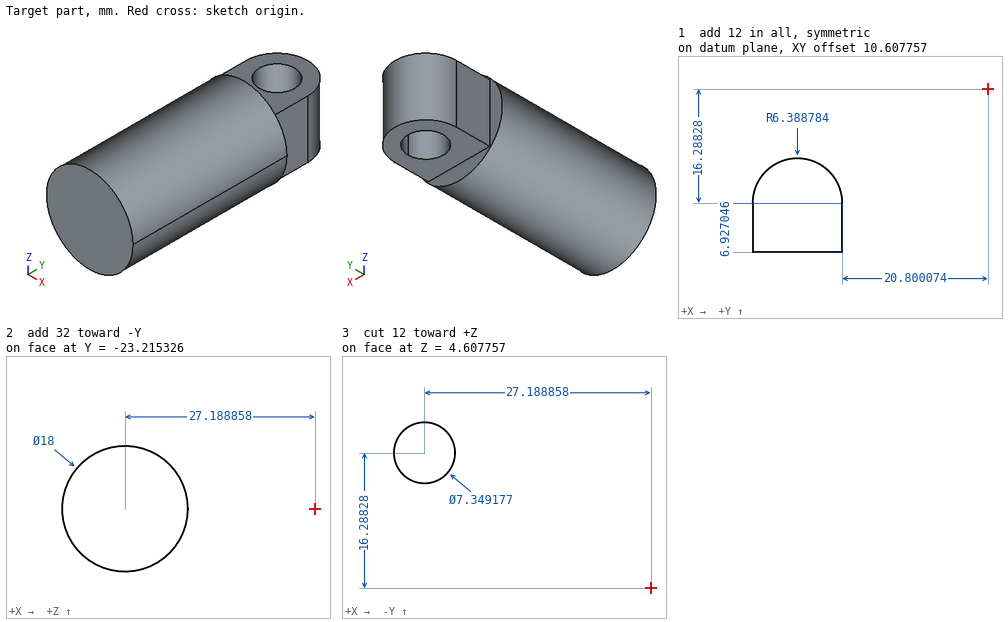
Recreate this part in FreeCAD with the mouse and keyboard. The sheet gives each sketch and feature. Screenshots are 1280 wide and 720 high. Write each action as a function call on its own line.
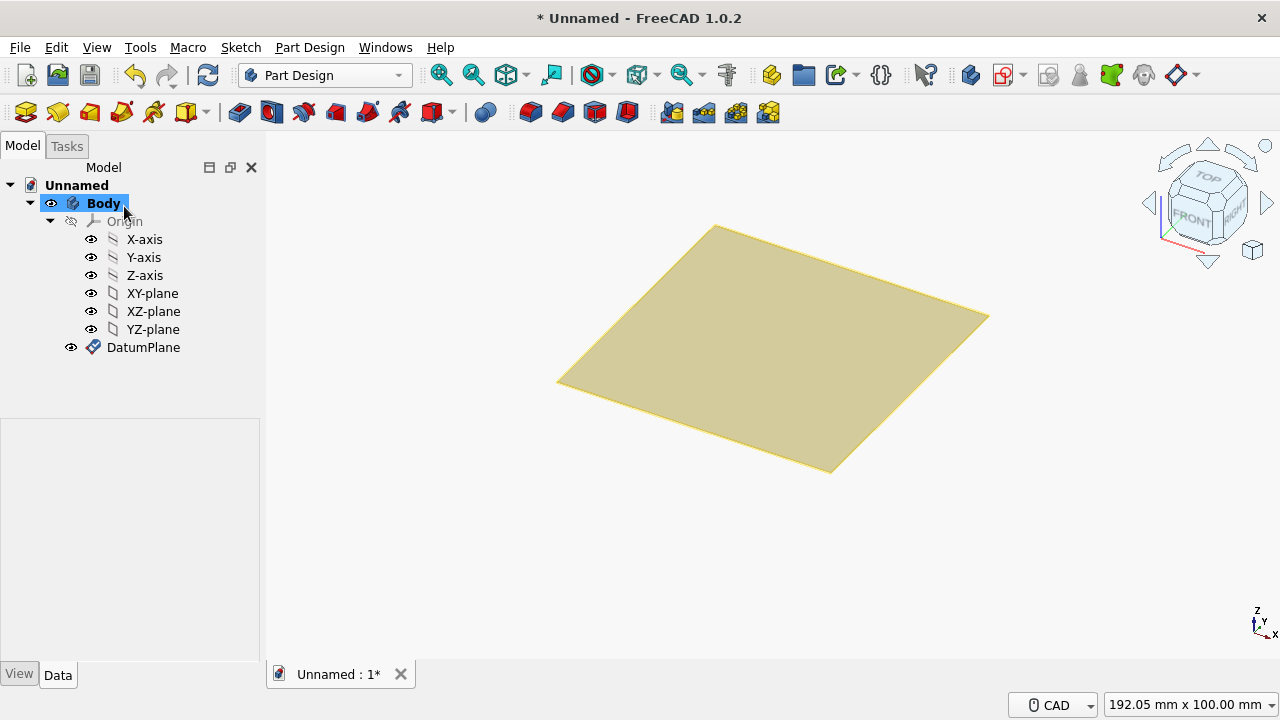
click(116, 347)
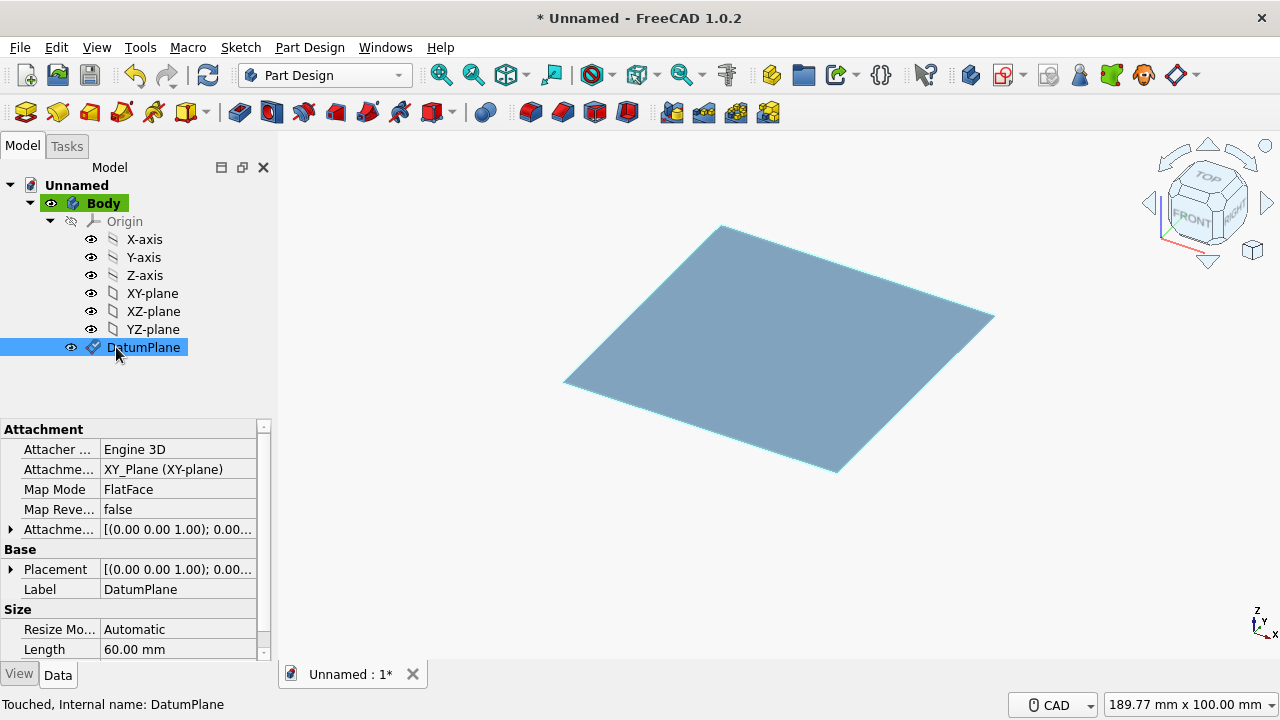
click(1004, 76)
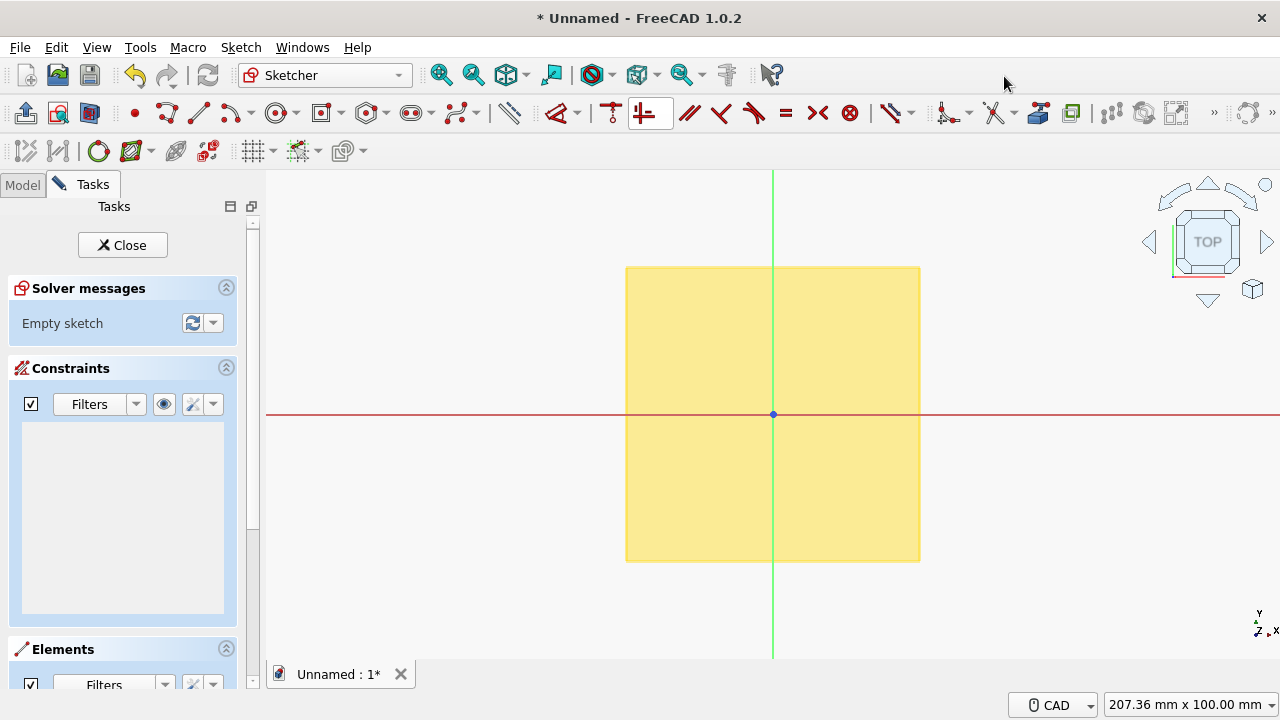
scroll(624, 516, up, 8)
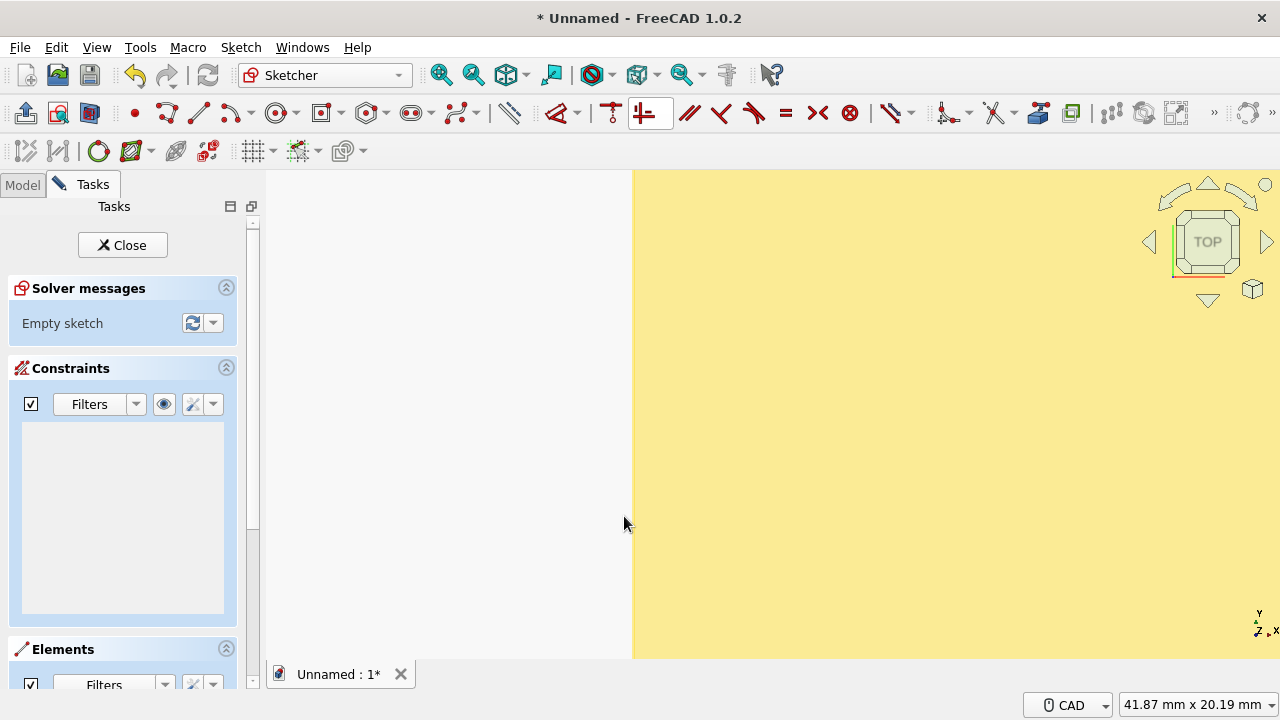
click(168, 114)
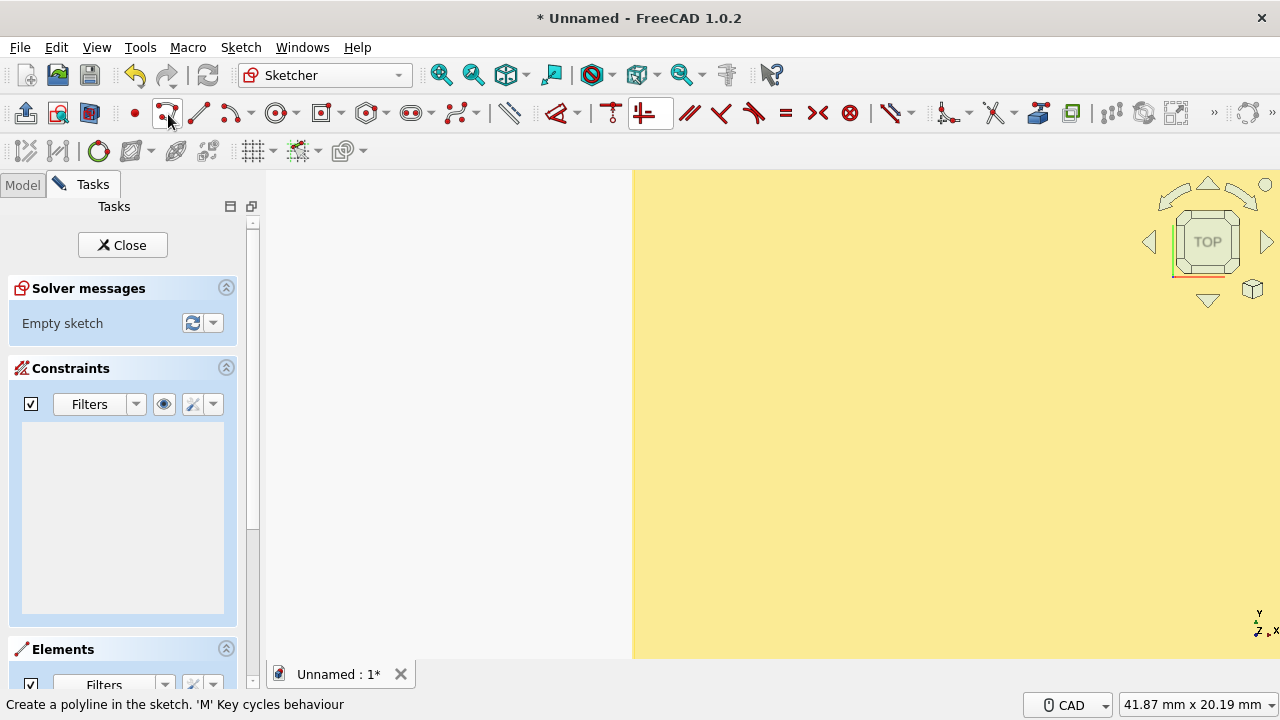
click(857, 405)
click(857, 573)
click(547, 573)
click(547, 405)
right_click(547, 405)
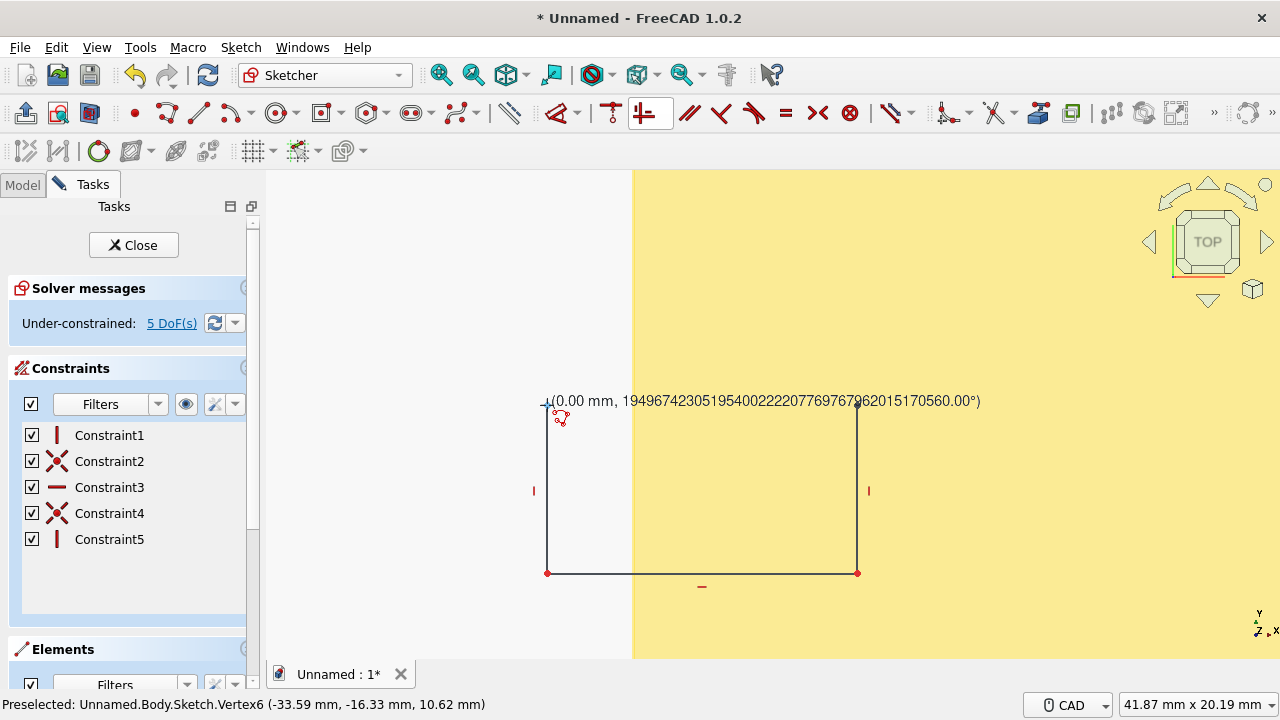
click(254, 114)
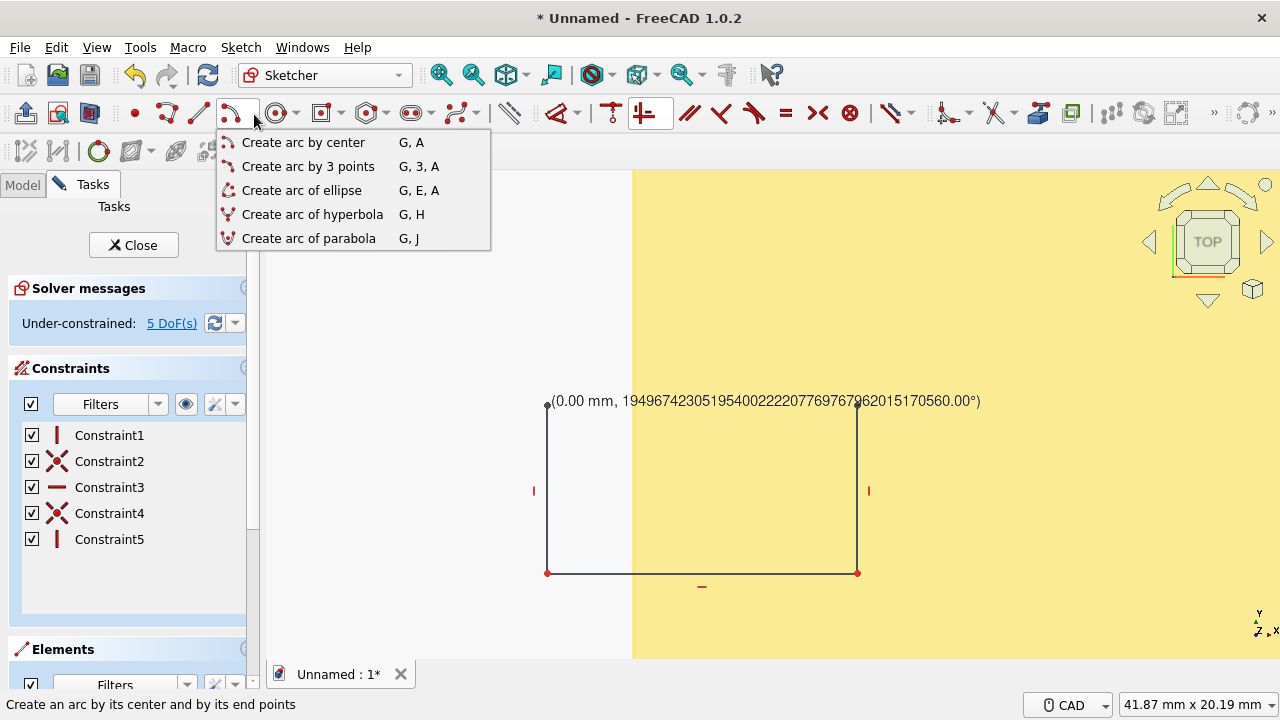
click(354, 166)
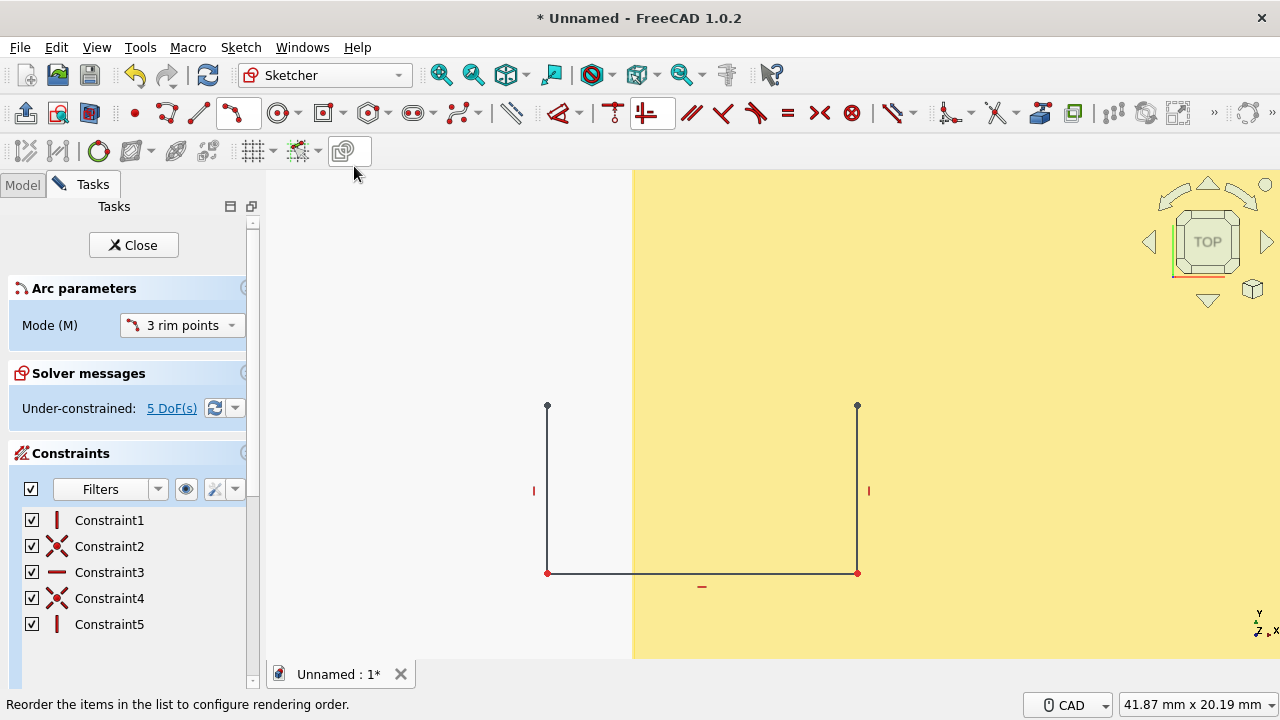
click(547, 406)
click(857, 406)
click(702, 250)
key(Escape)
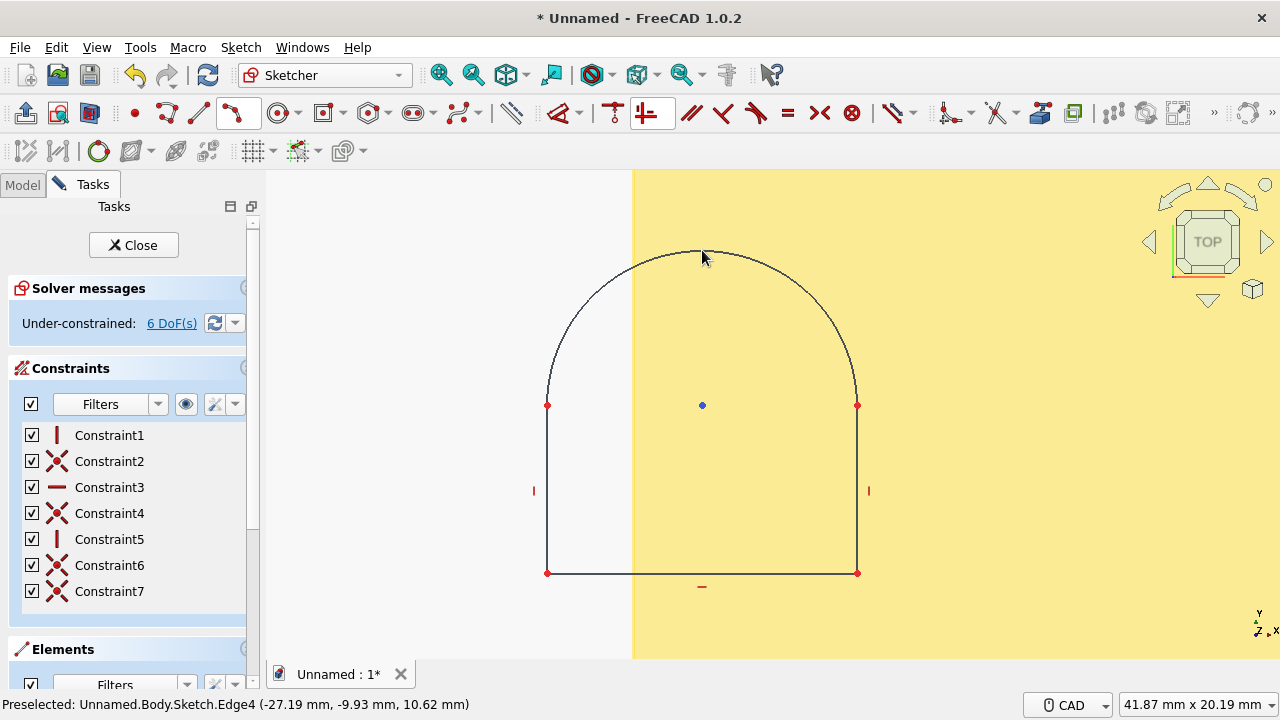
click(857, 456)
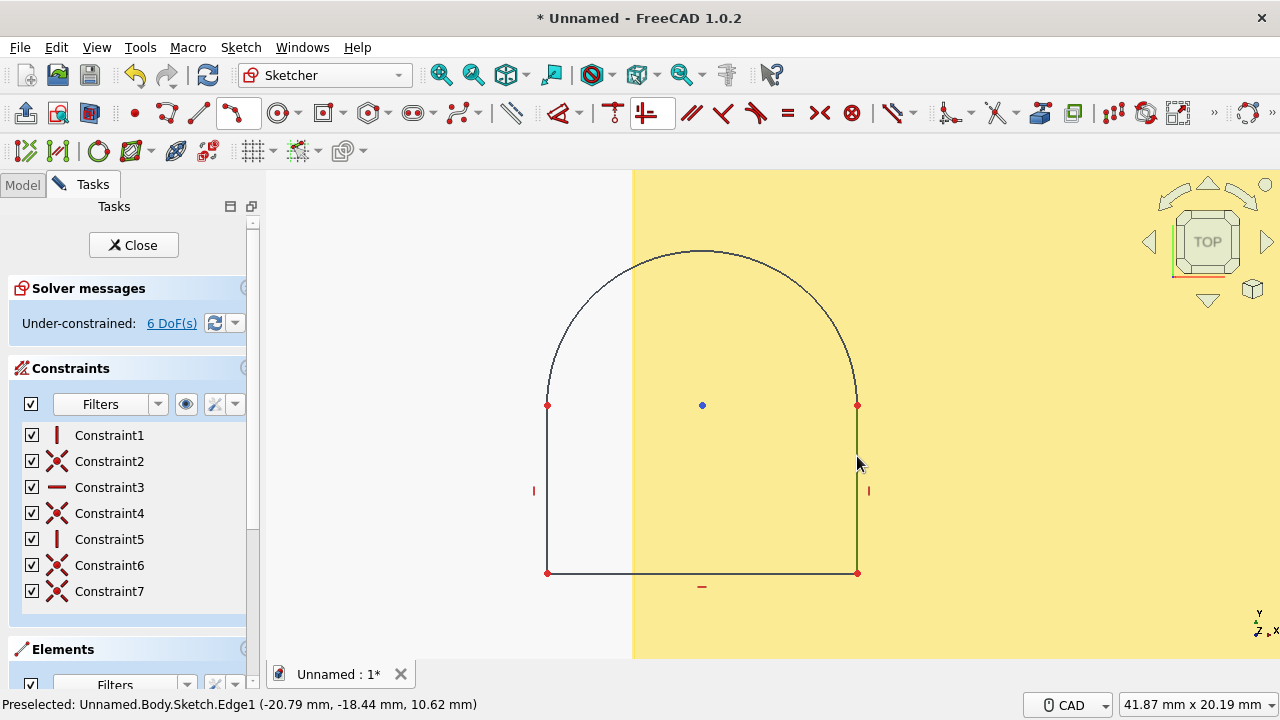
click(793, 281)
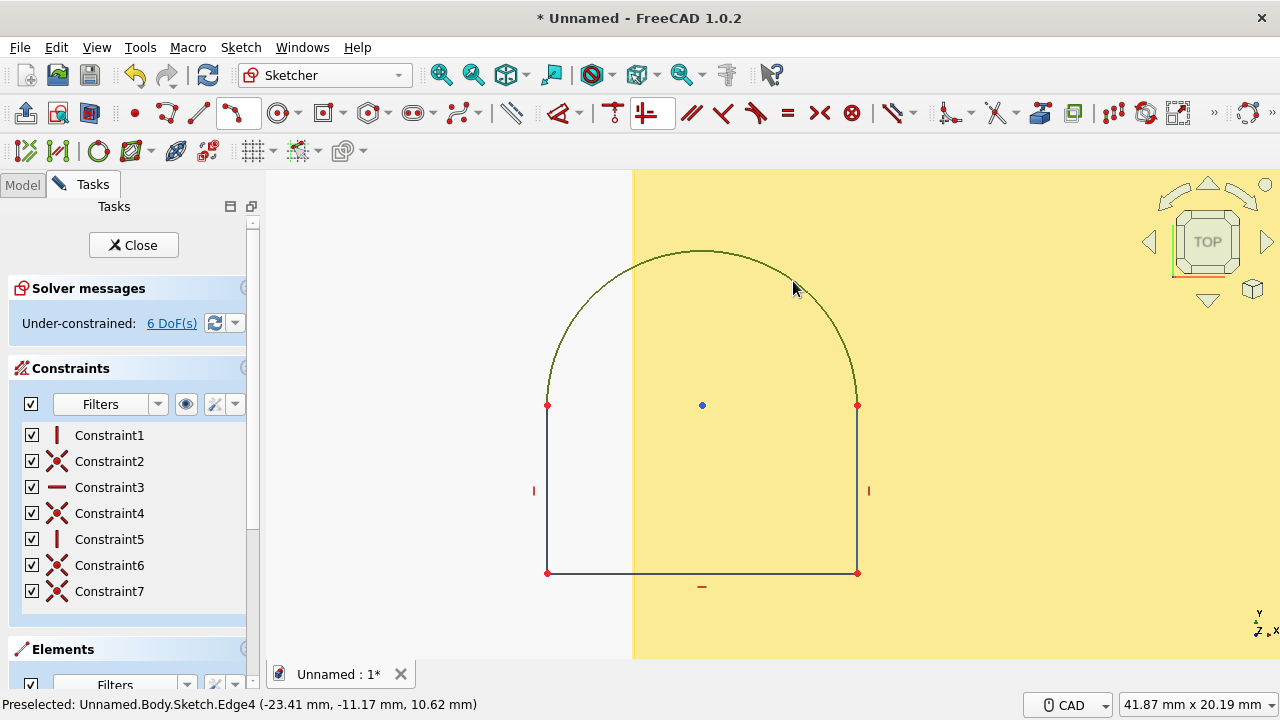
click(756, 114)